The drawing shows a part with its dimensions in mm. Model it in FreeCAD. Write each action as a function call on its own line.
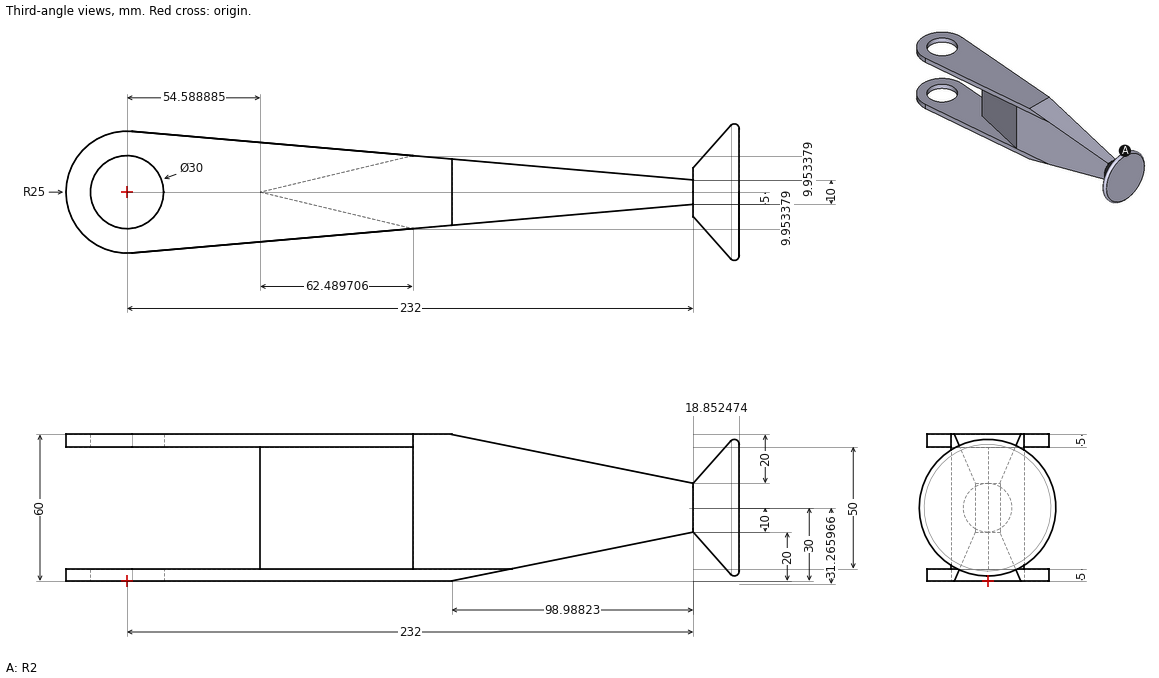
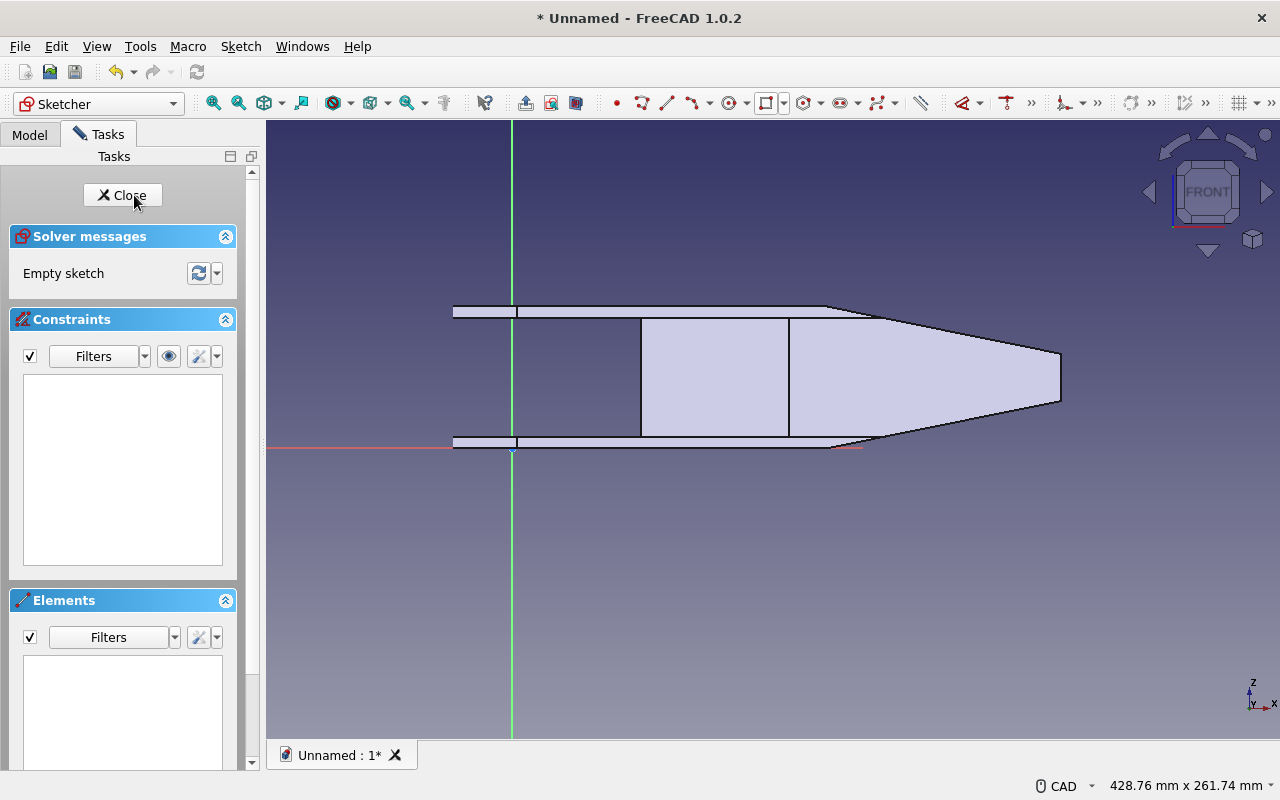
click(576, 104)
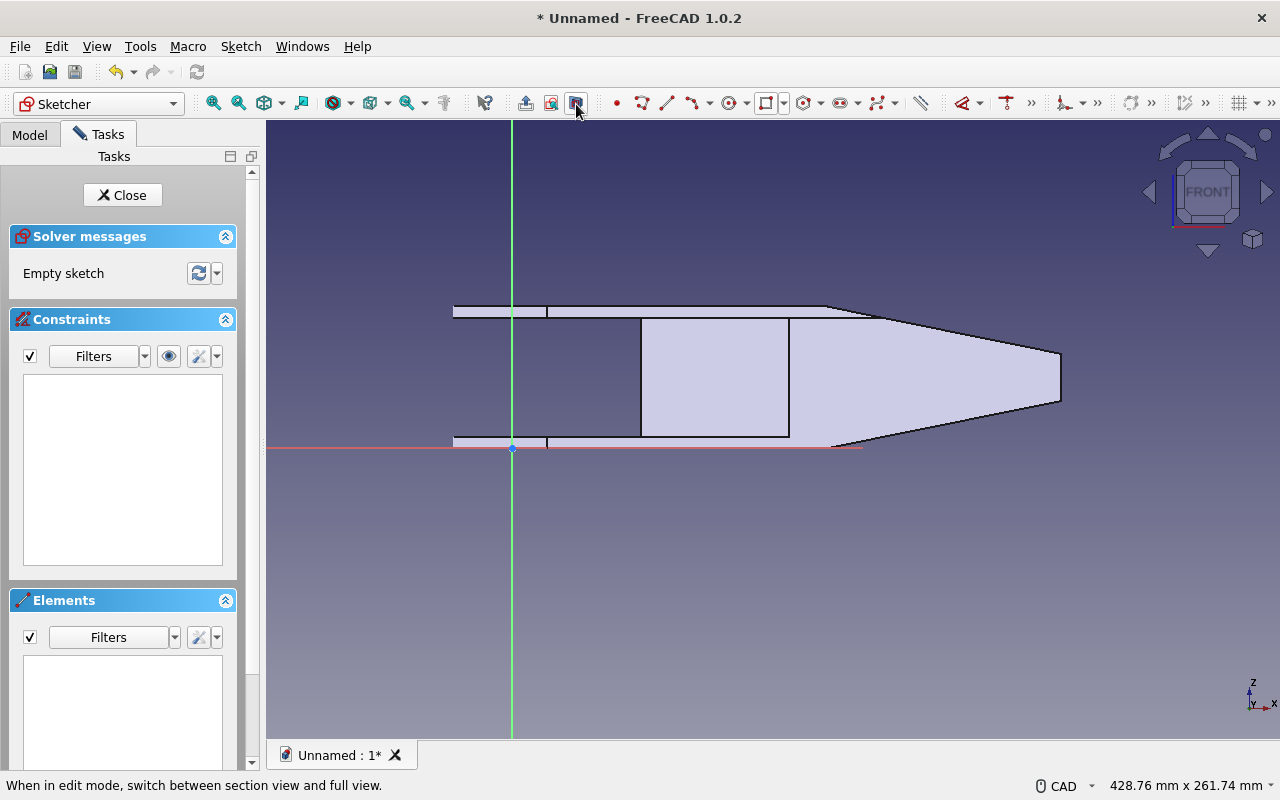
scroll(1115, 411, up, 8)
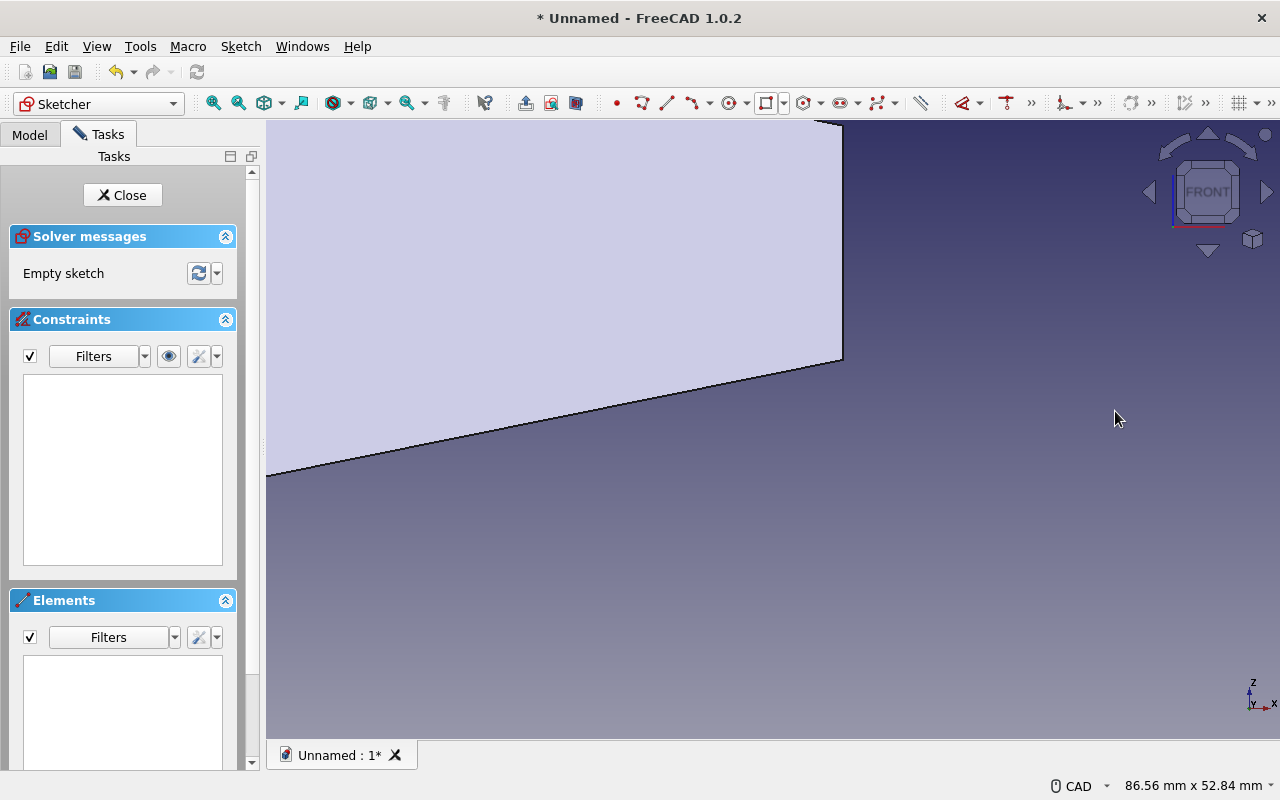
click(642, 104)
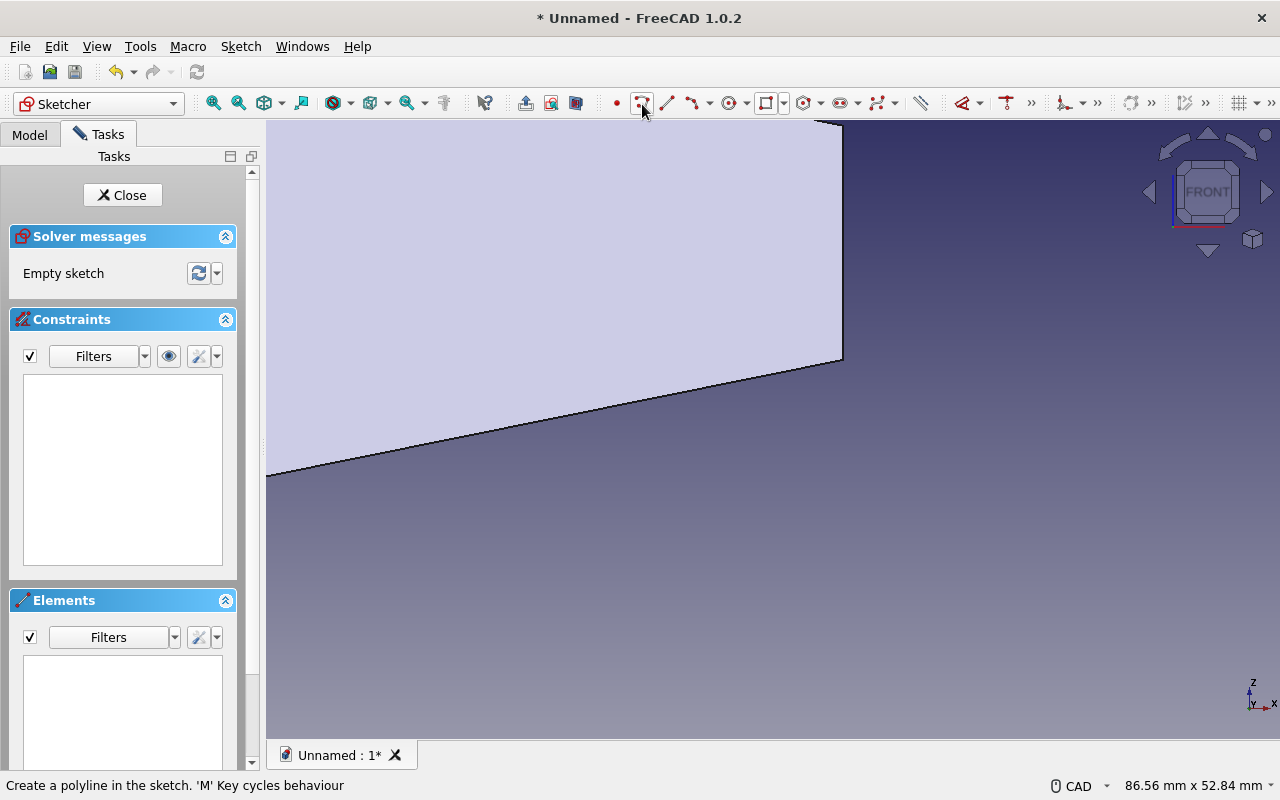
click(843, 360)
click(843, 243)
click(1064, 243)
click(1064, 609)
click(843, 361)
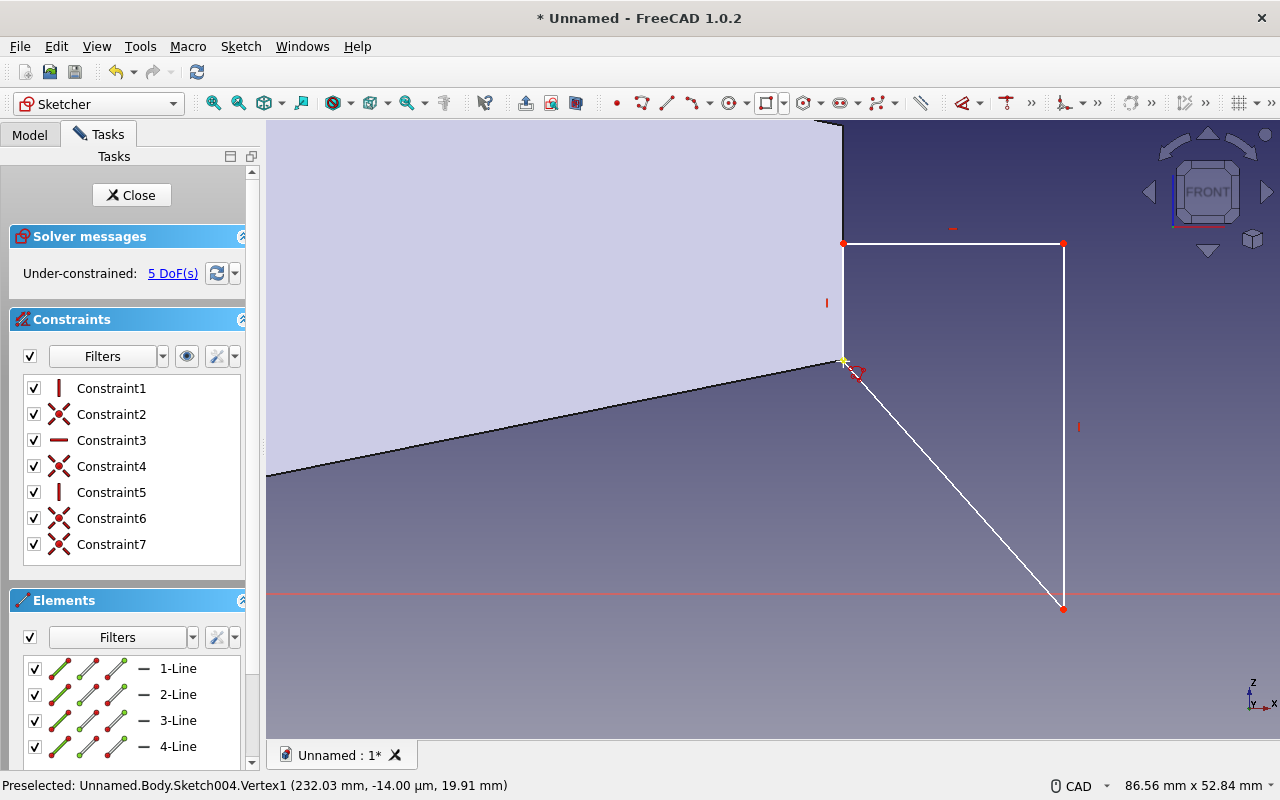
click(667, 104)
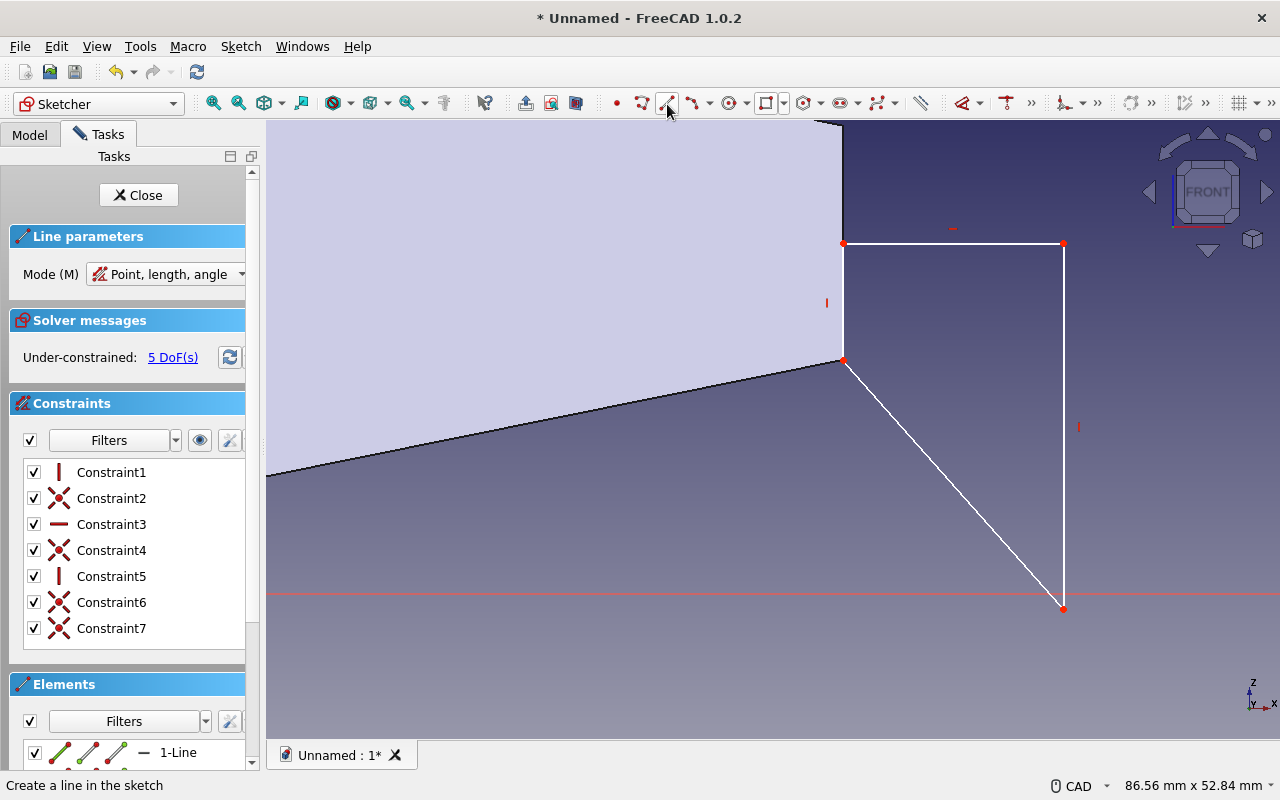
click(821, 243)
click(754, 243)
key(Escape)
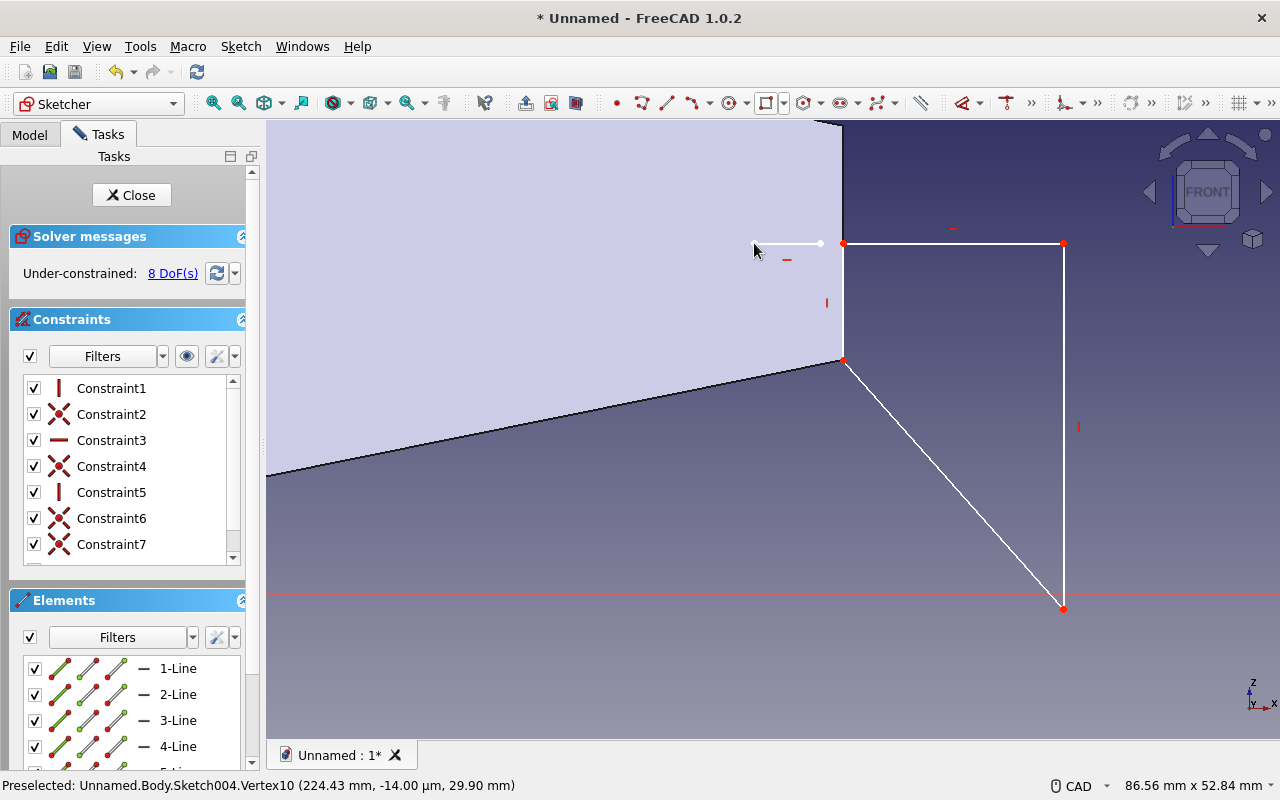
click(801, 244)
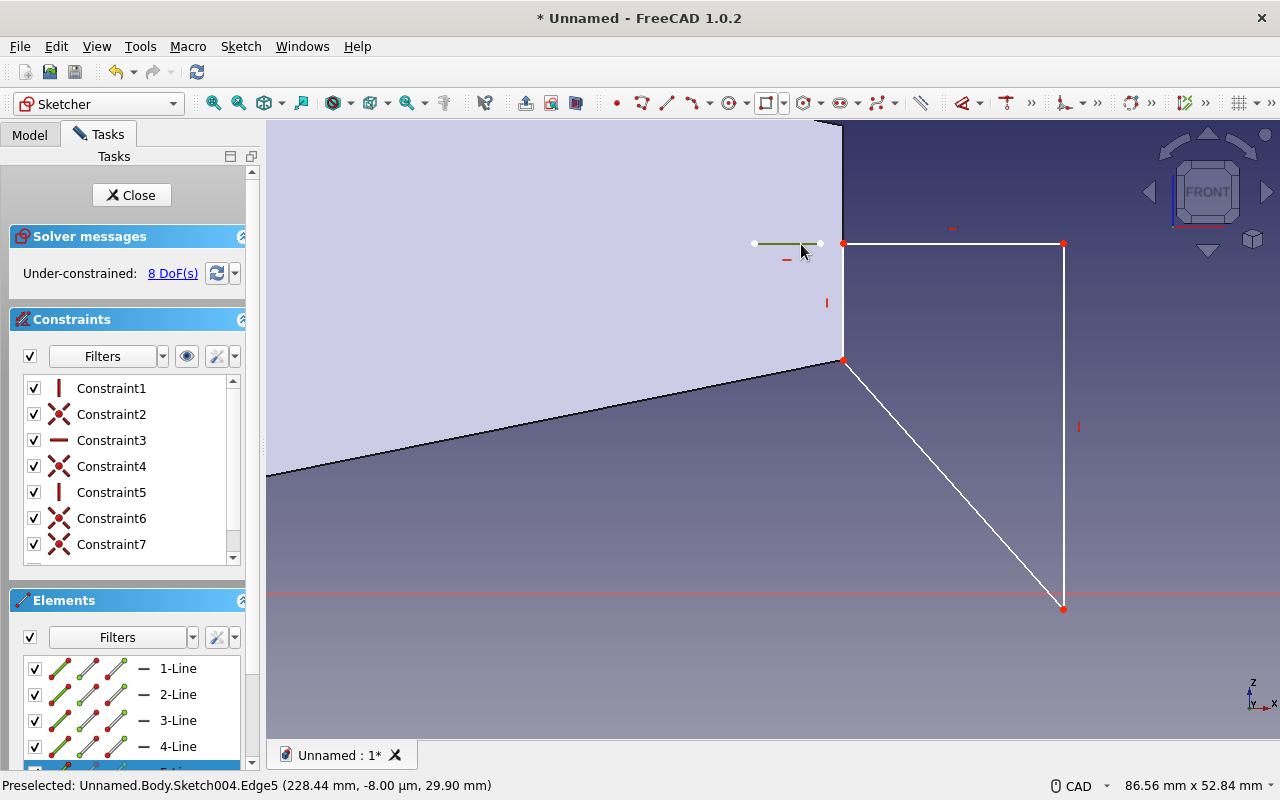
click(921, 104)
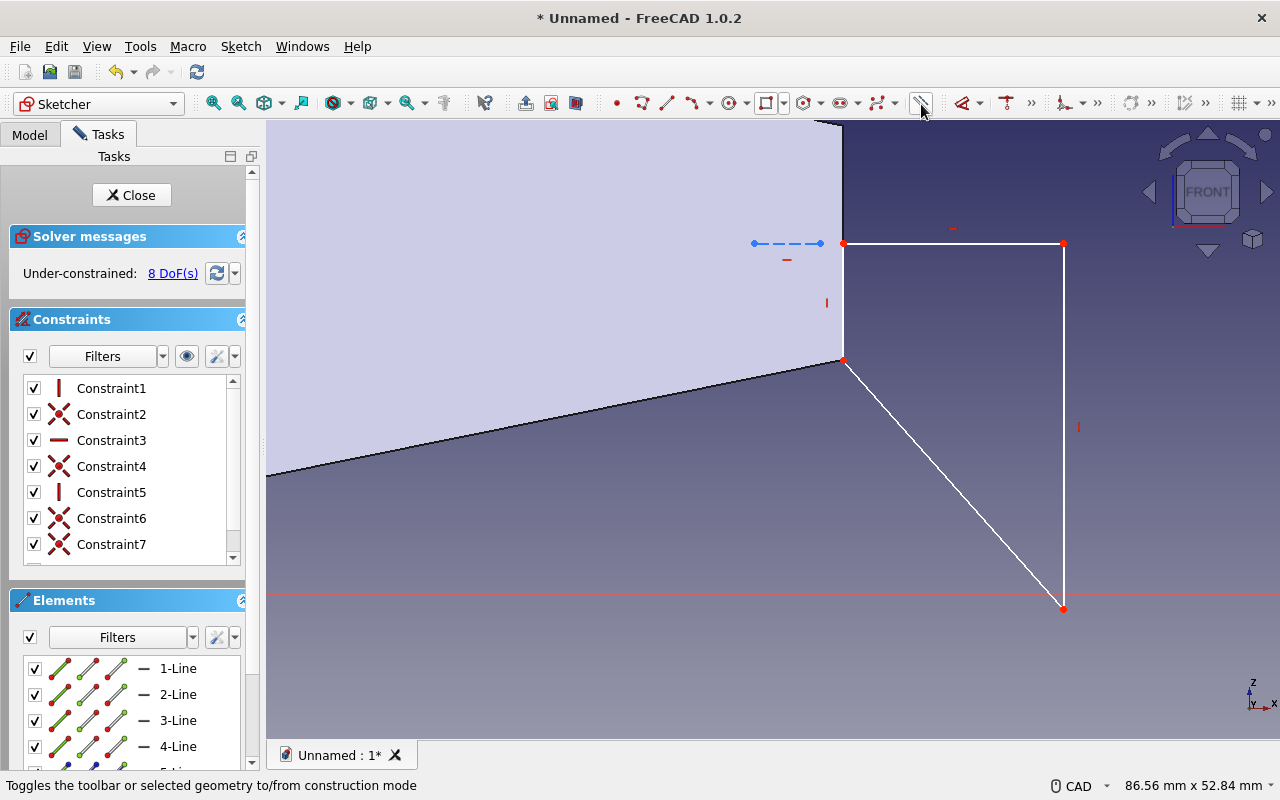
click(962, 104)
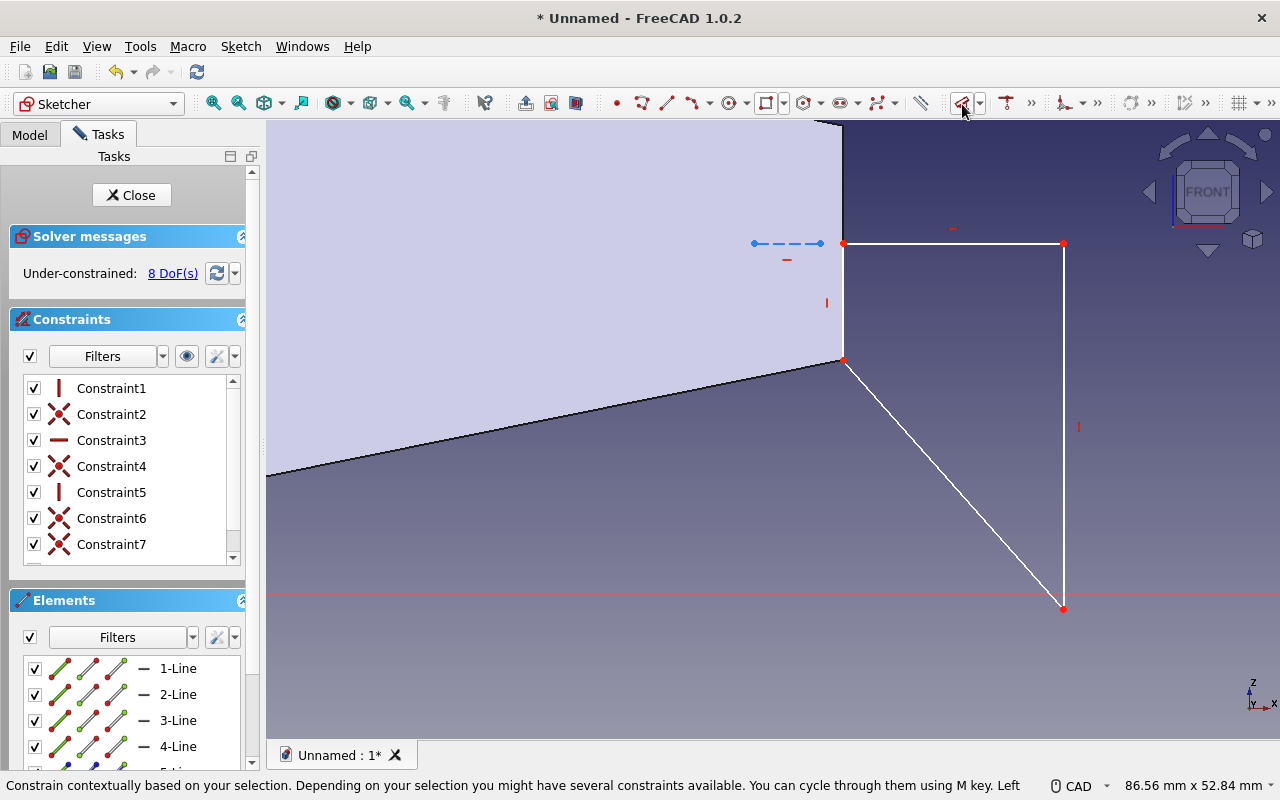
click(843, 326)
click(809, 303)